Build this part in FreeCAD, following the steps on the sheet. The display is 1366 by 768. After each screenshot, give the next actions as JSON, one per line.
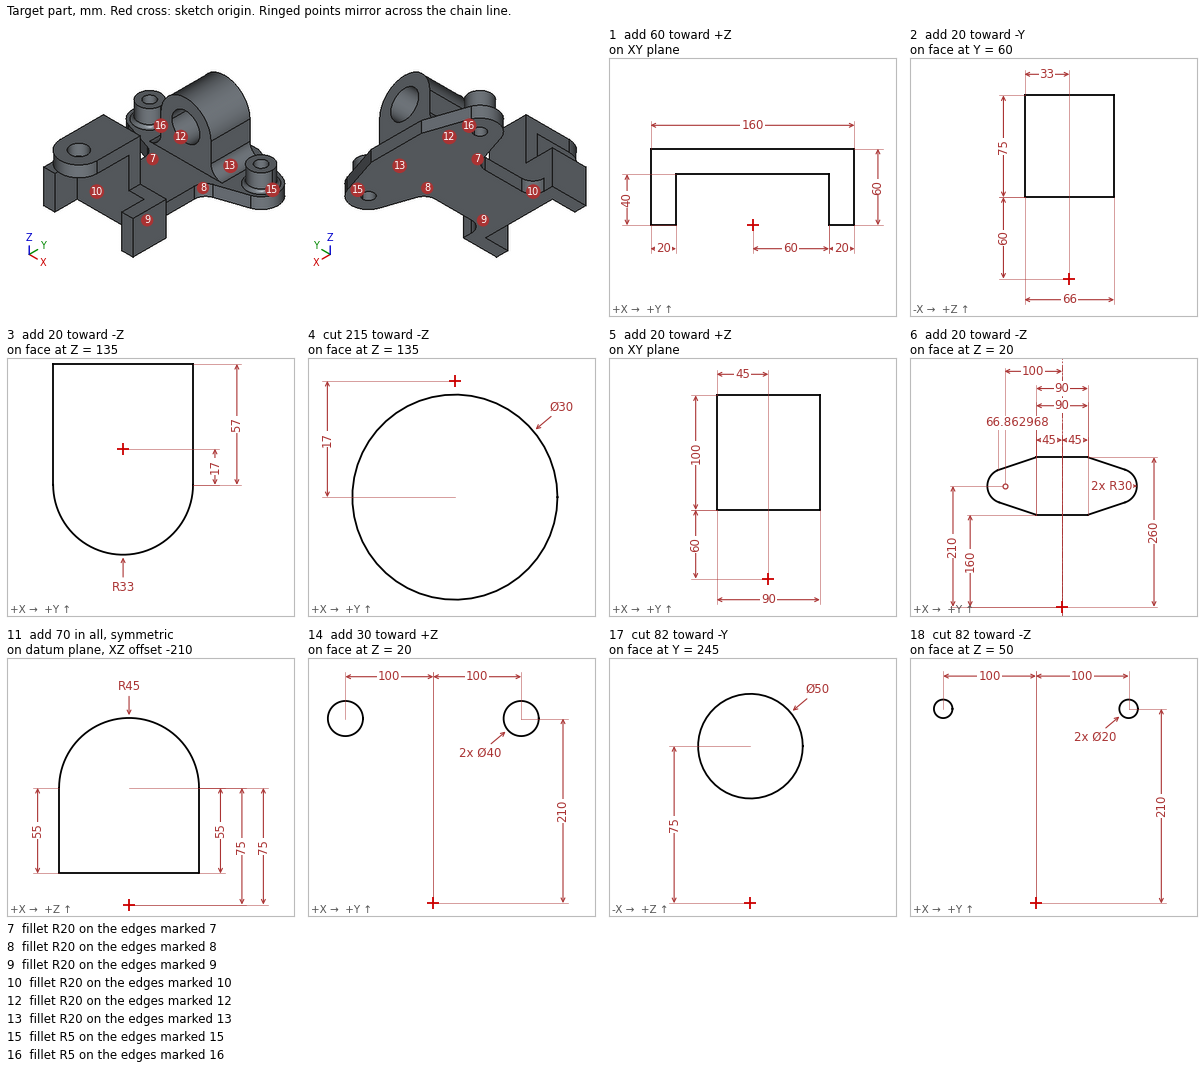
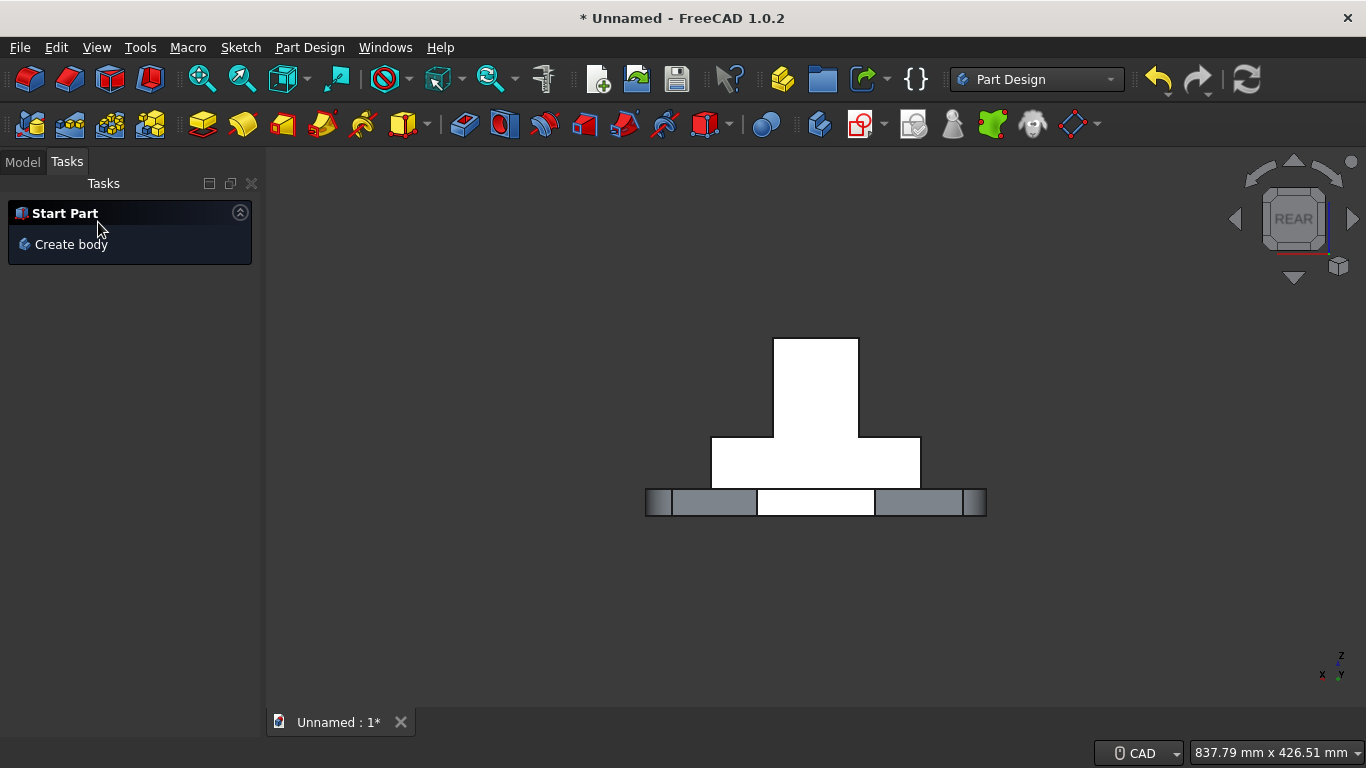
{"action": "key", "text": "6"}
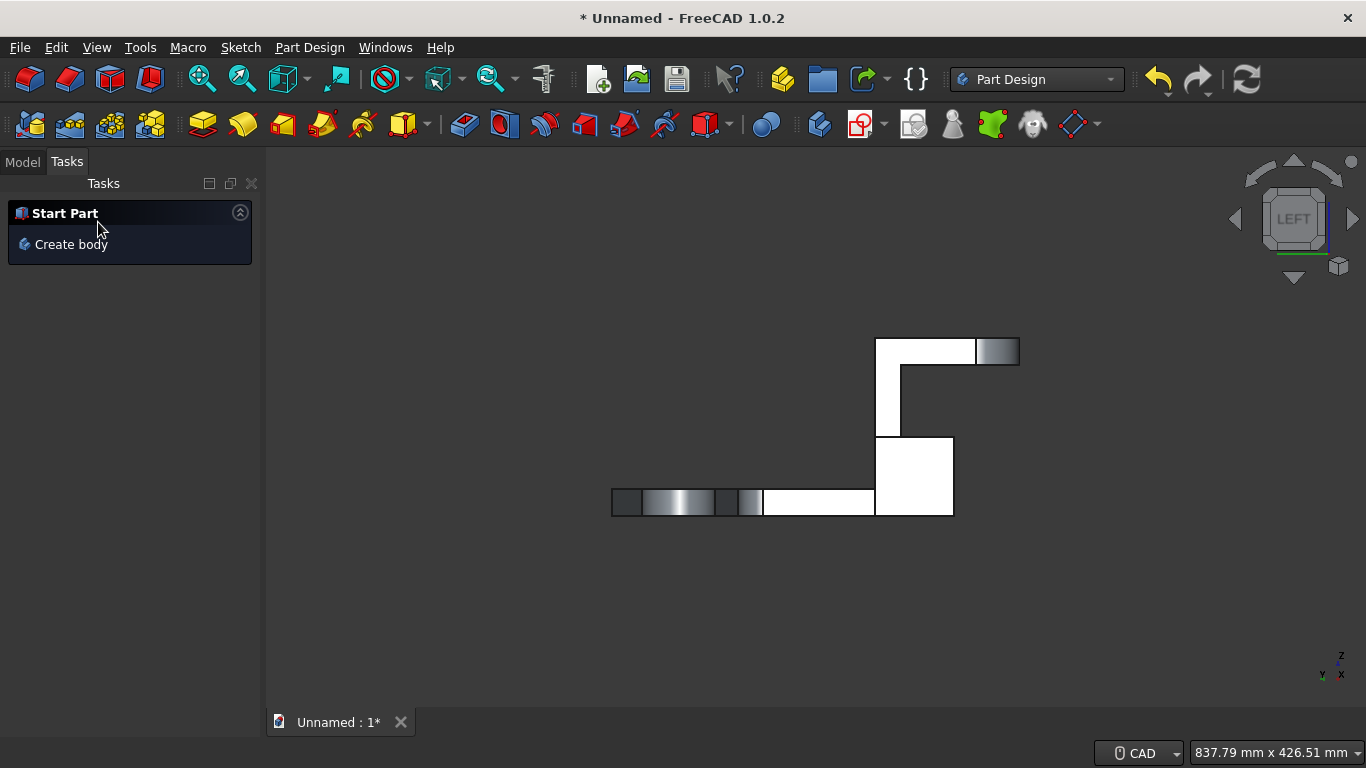
{"action": "key", "text": "v f"}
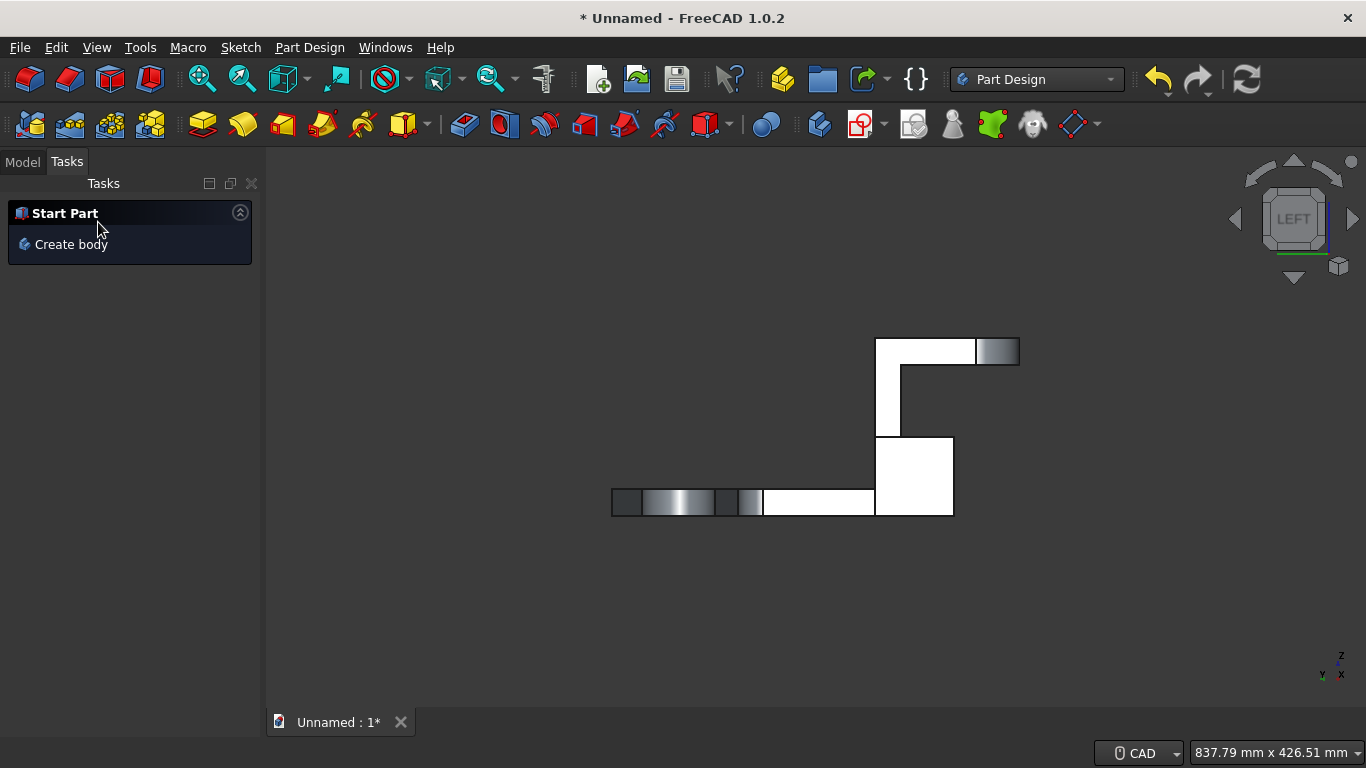
{"action": "key", "text": "v 3"}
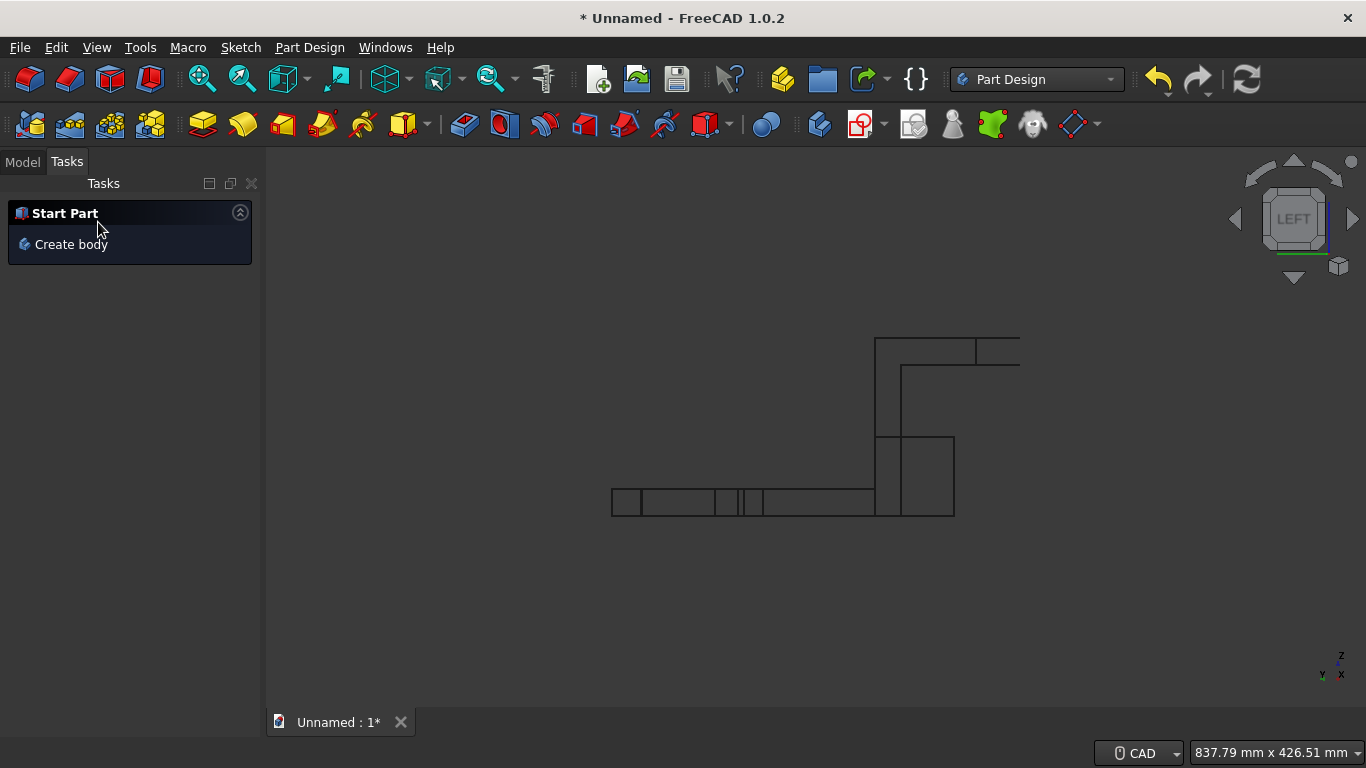
{"action": "key", "text": "0"}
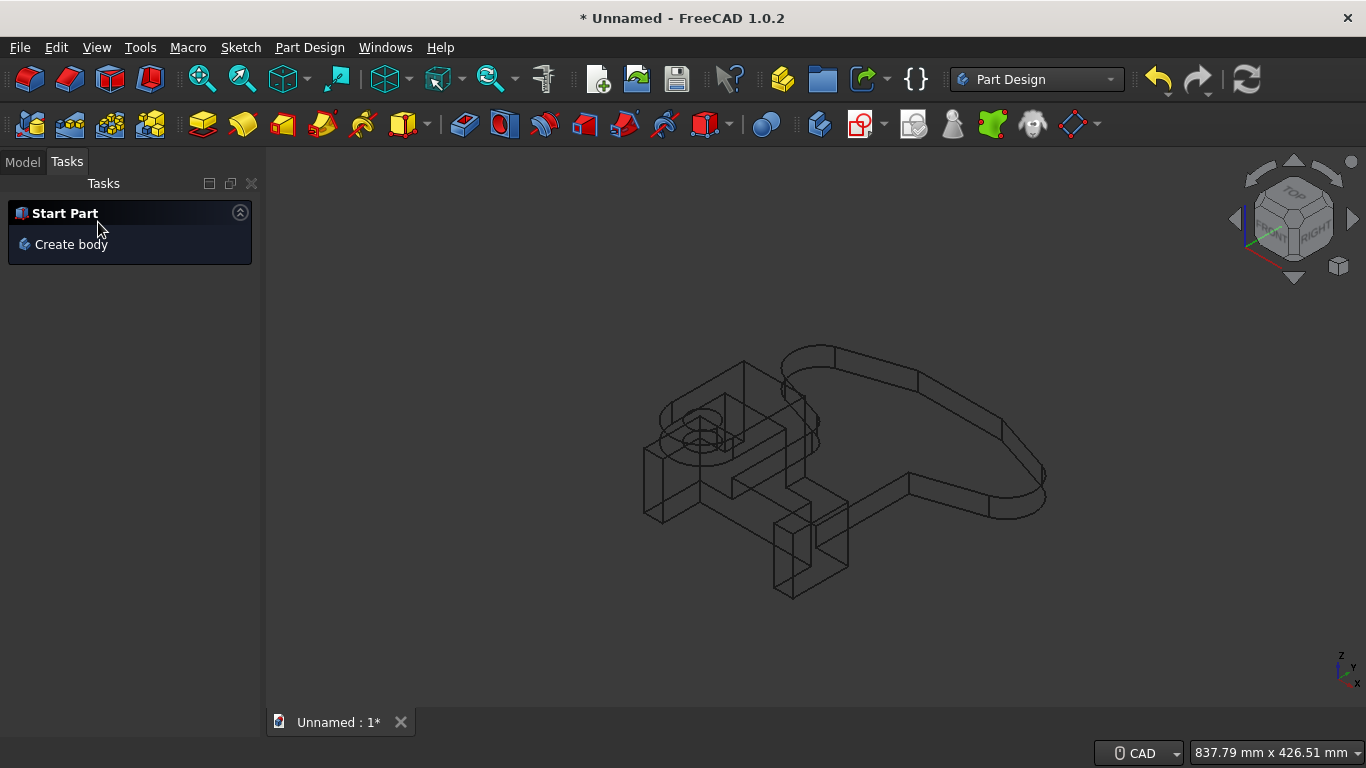
{"action": "left_click", "coordinate": [909, 482]}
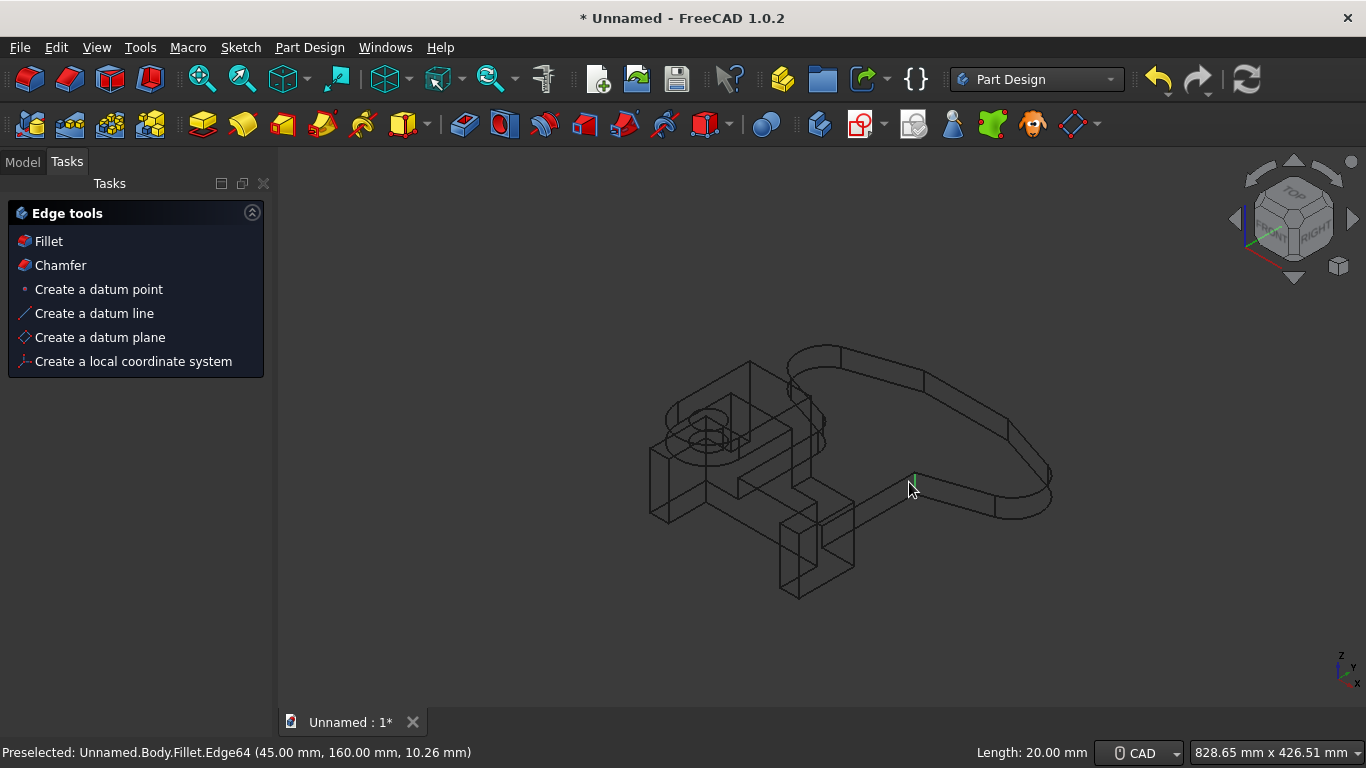
{"action": "key", "text": "v 1"}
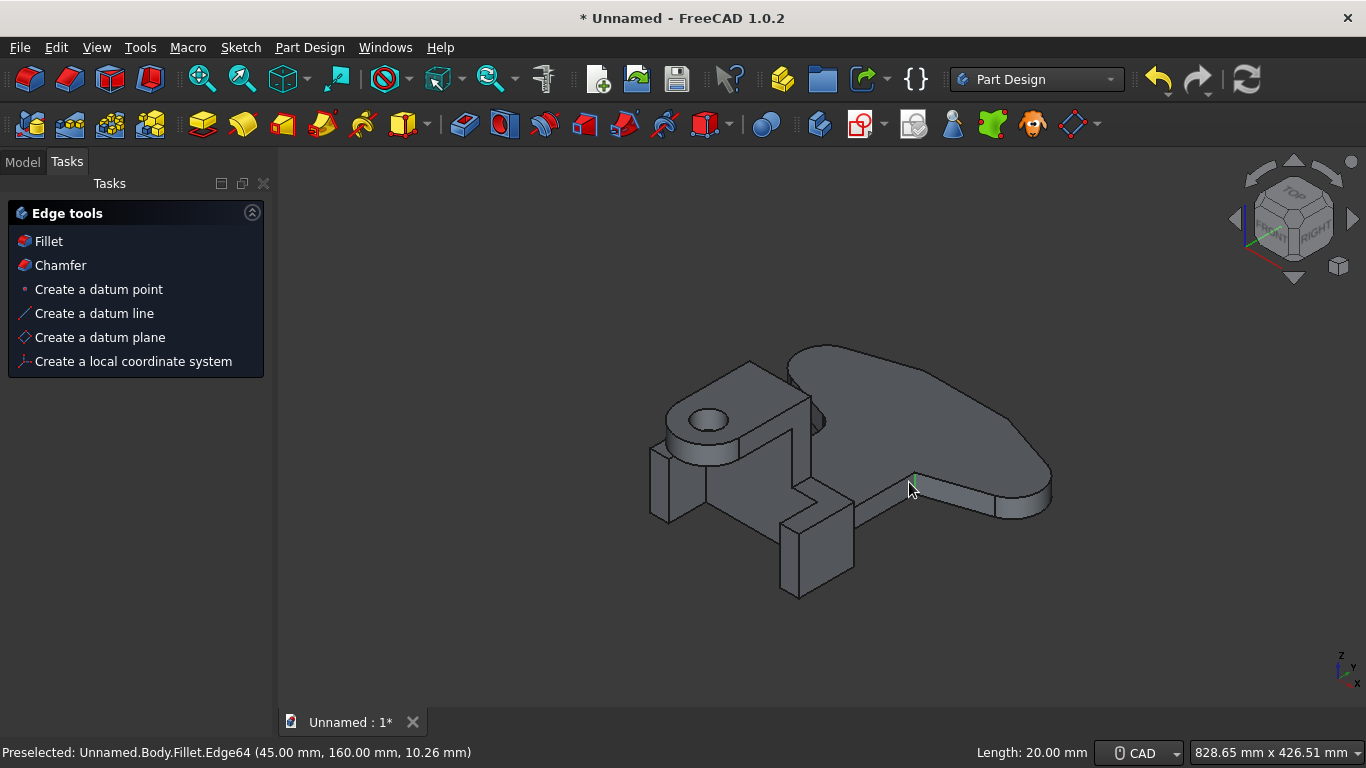
{"action": "left_click", "coordinate": [30, 80]}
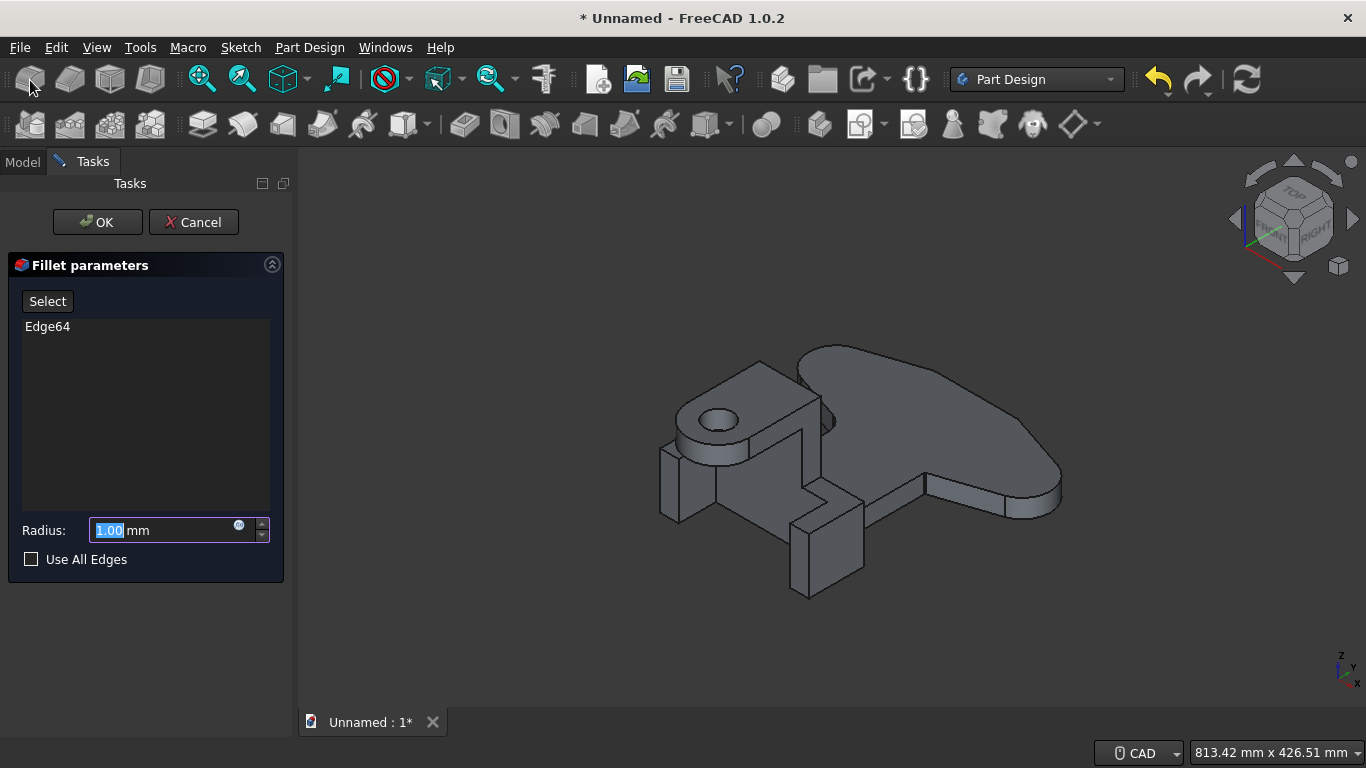
{"action": "type", "text": "20"}
{"action": "key", "text": "Tab"}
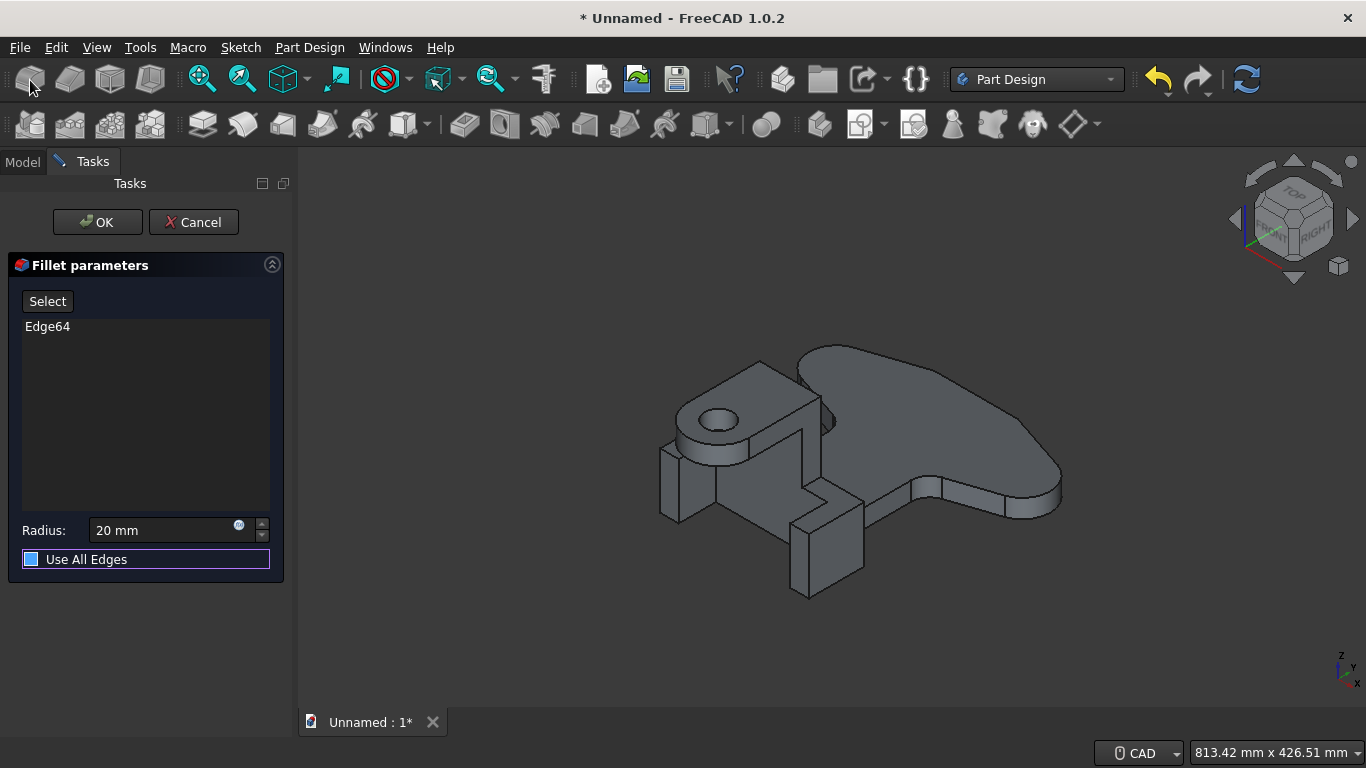
{"action": "left_click", "coordinate": [98, 222]}